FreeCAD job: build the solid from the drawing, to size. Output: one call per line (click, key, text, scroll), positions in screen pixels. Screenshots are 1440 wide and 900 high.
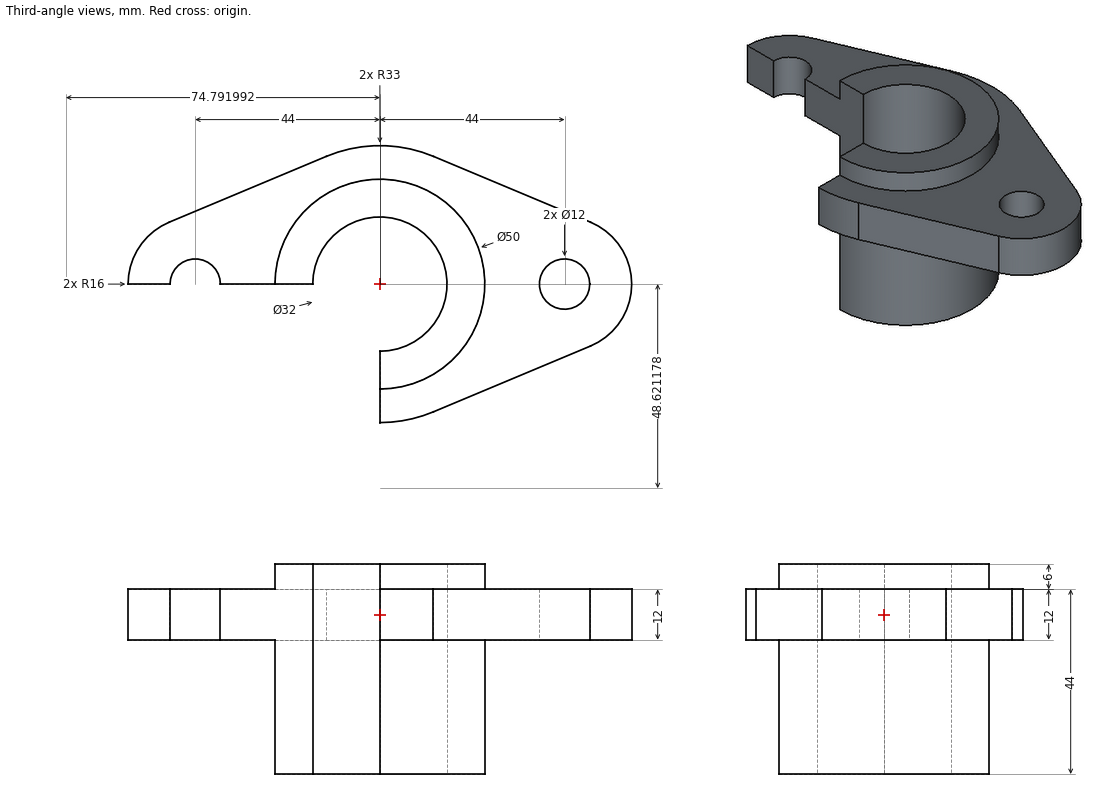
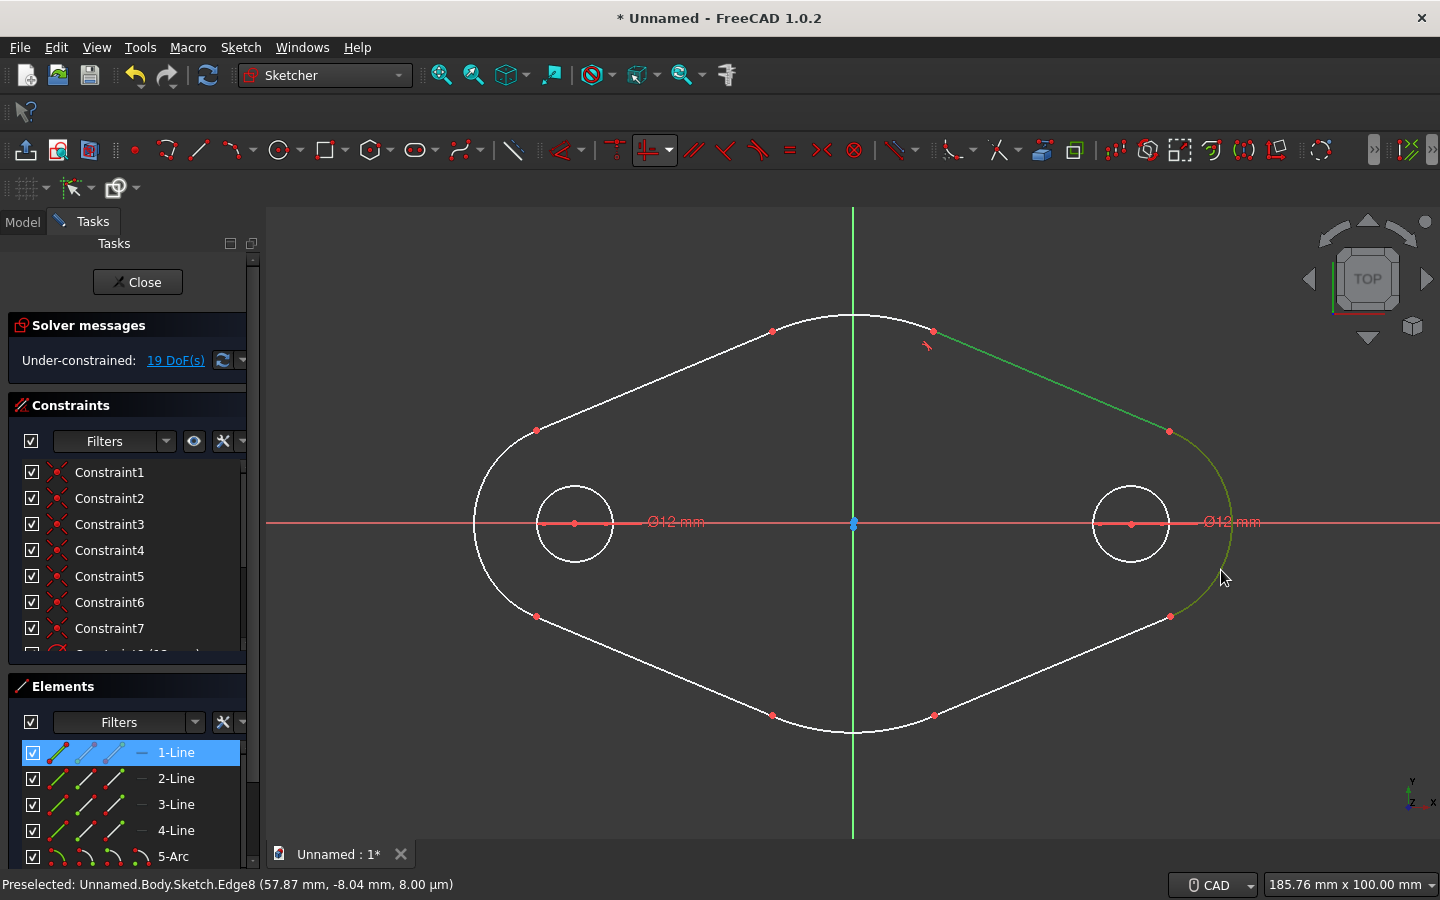
key(t)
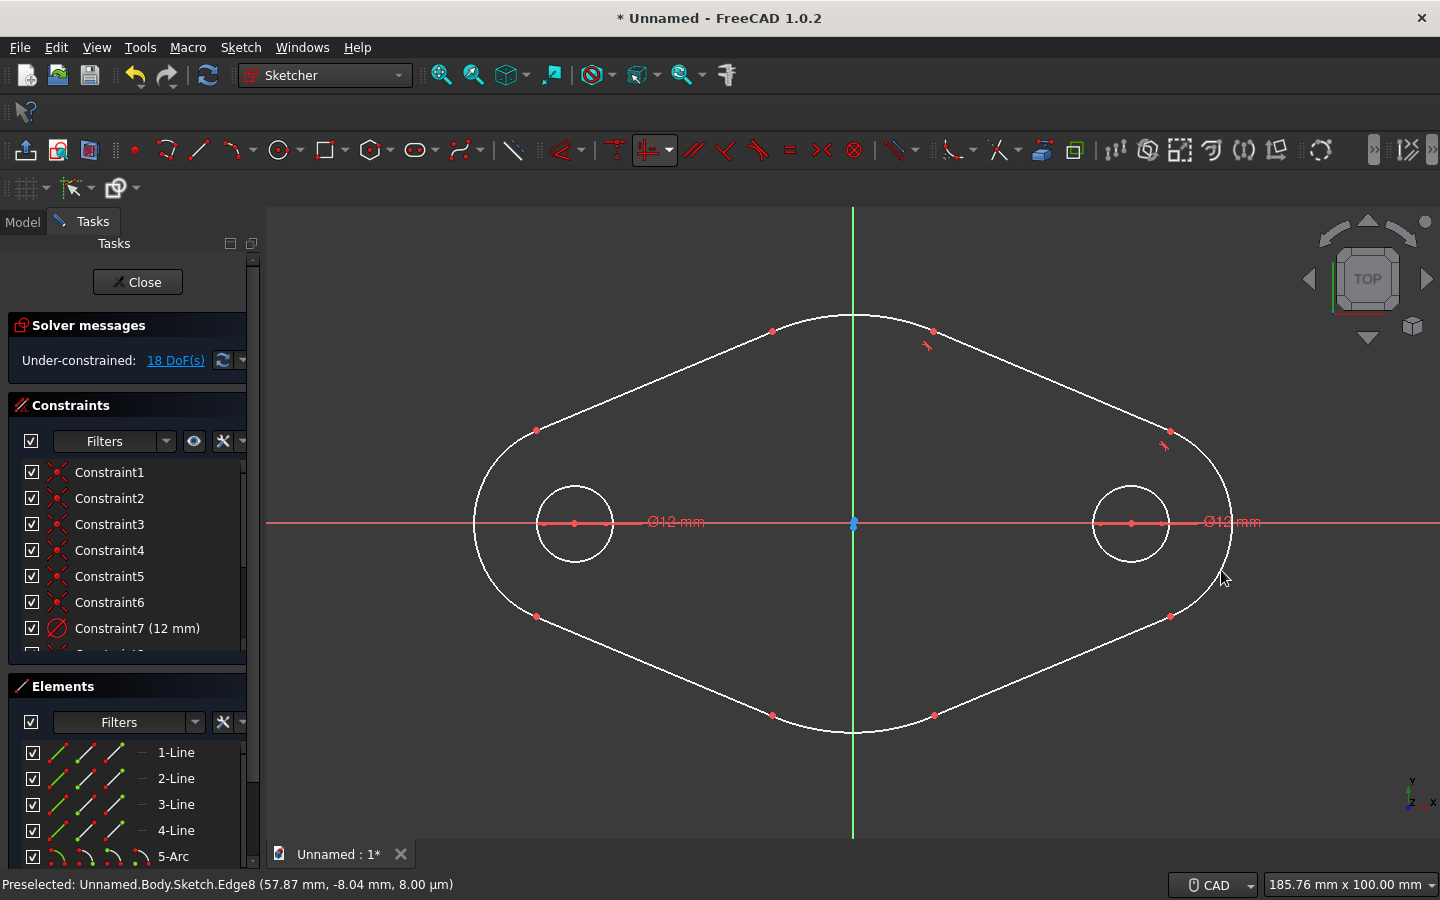
click(701, 362)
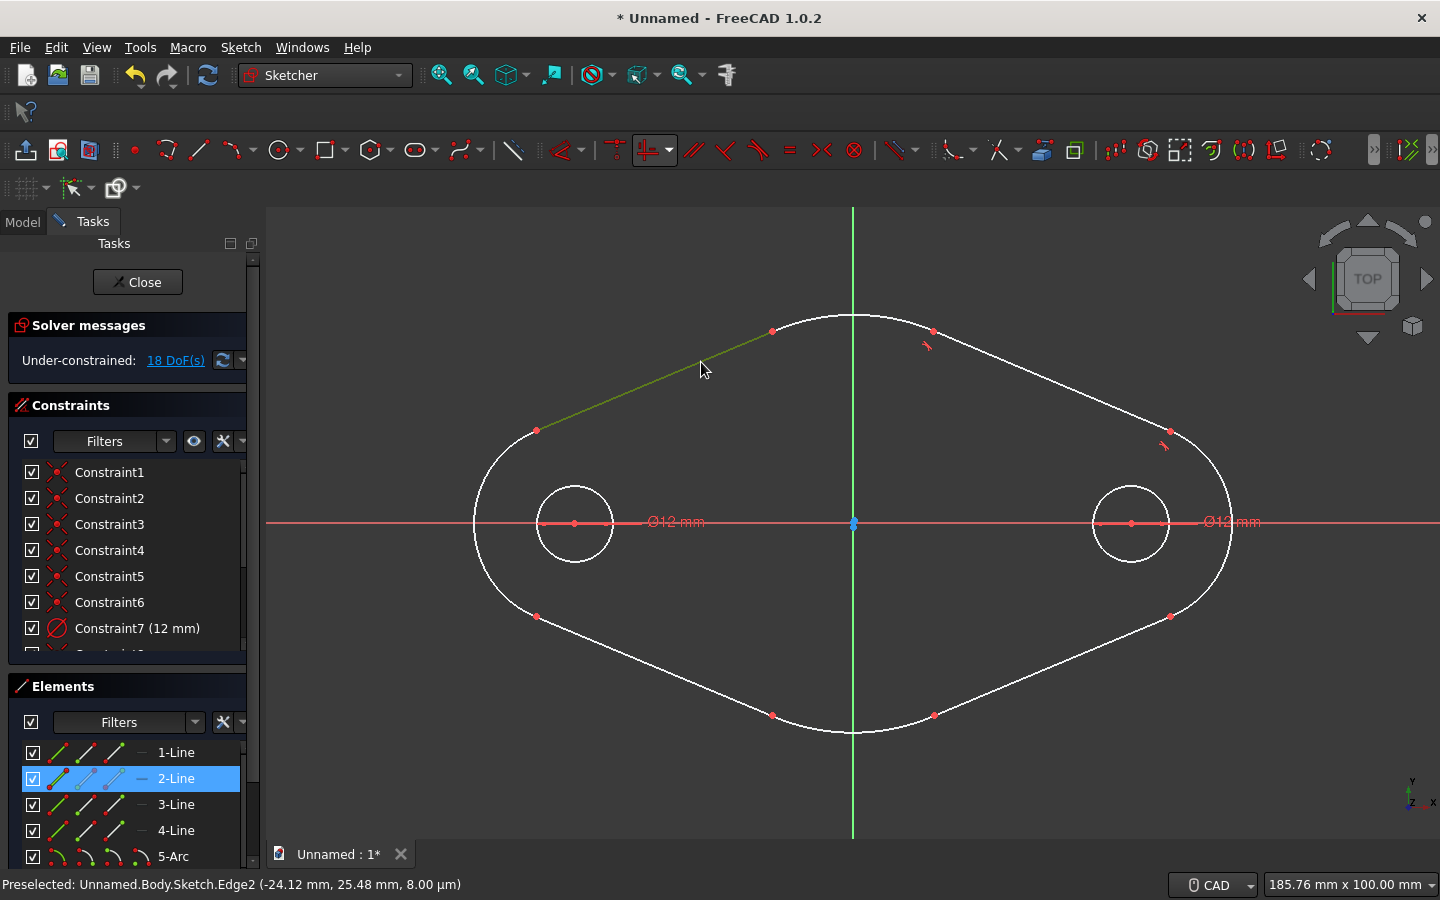
click(886, 317)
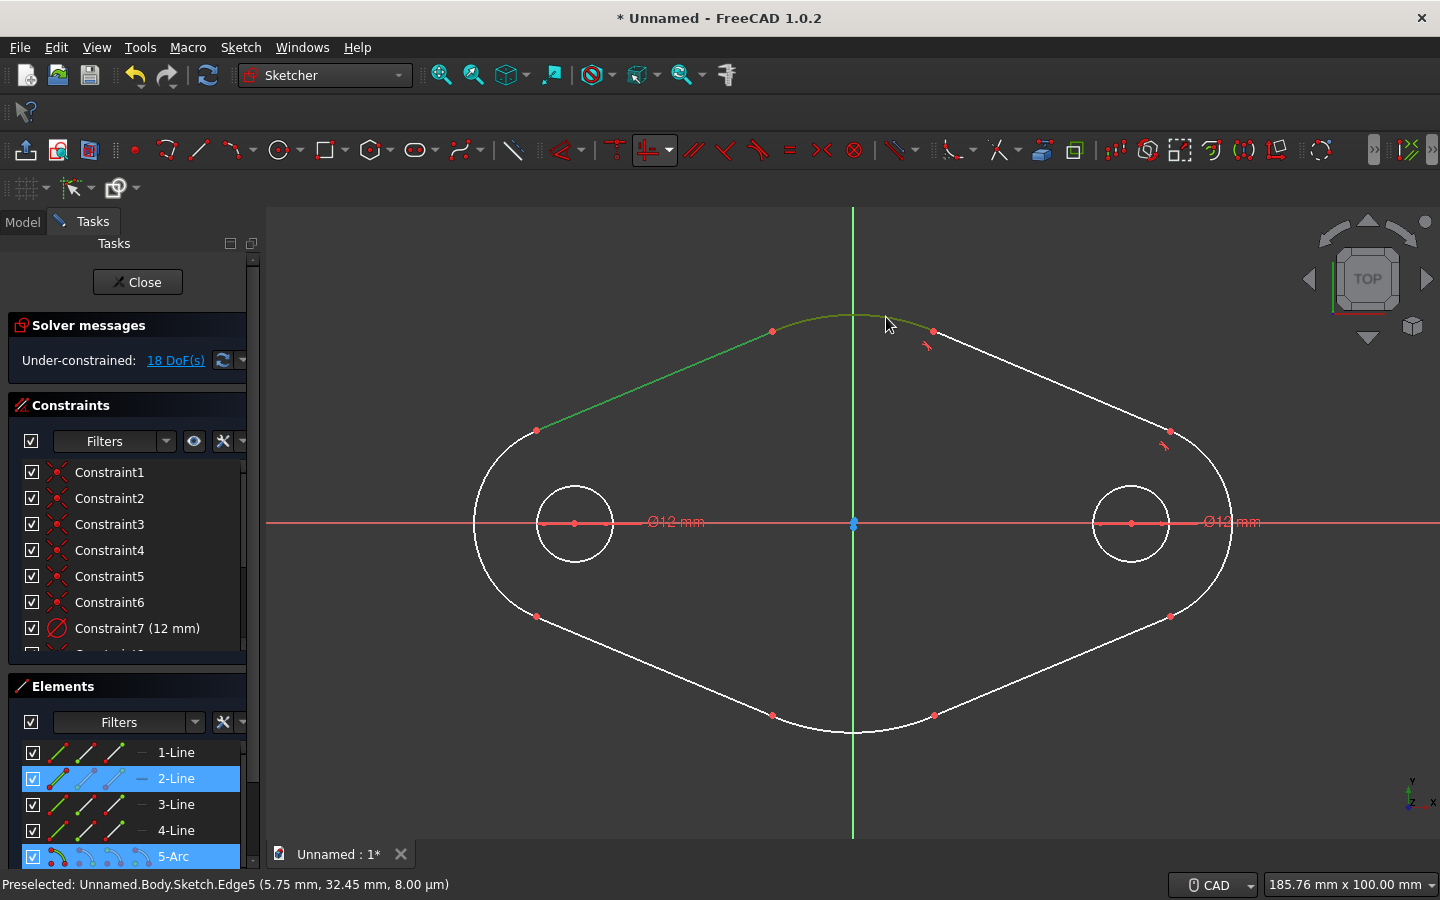
click(758, 150)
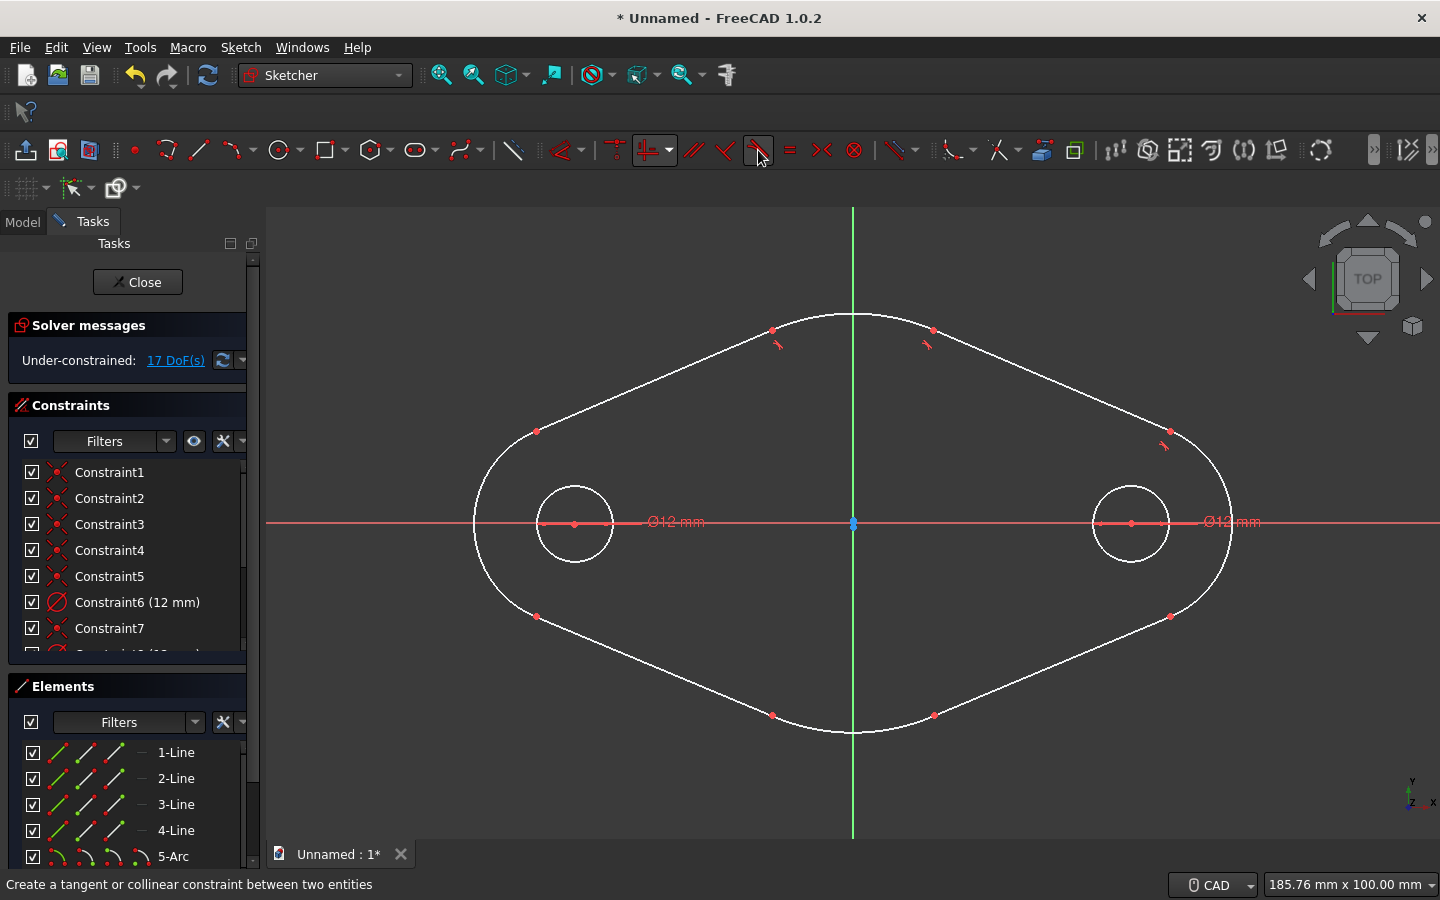
click(701, 360)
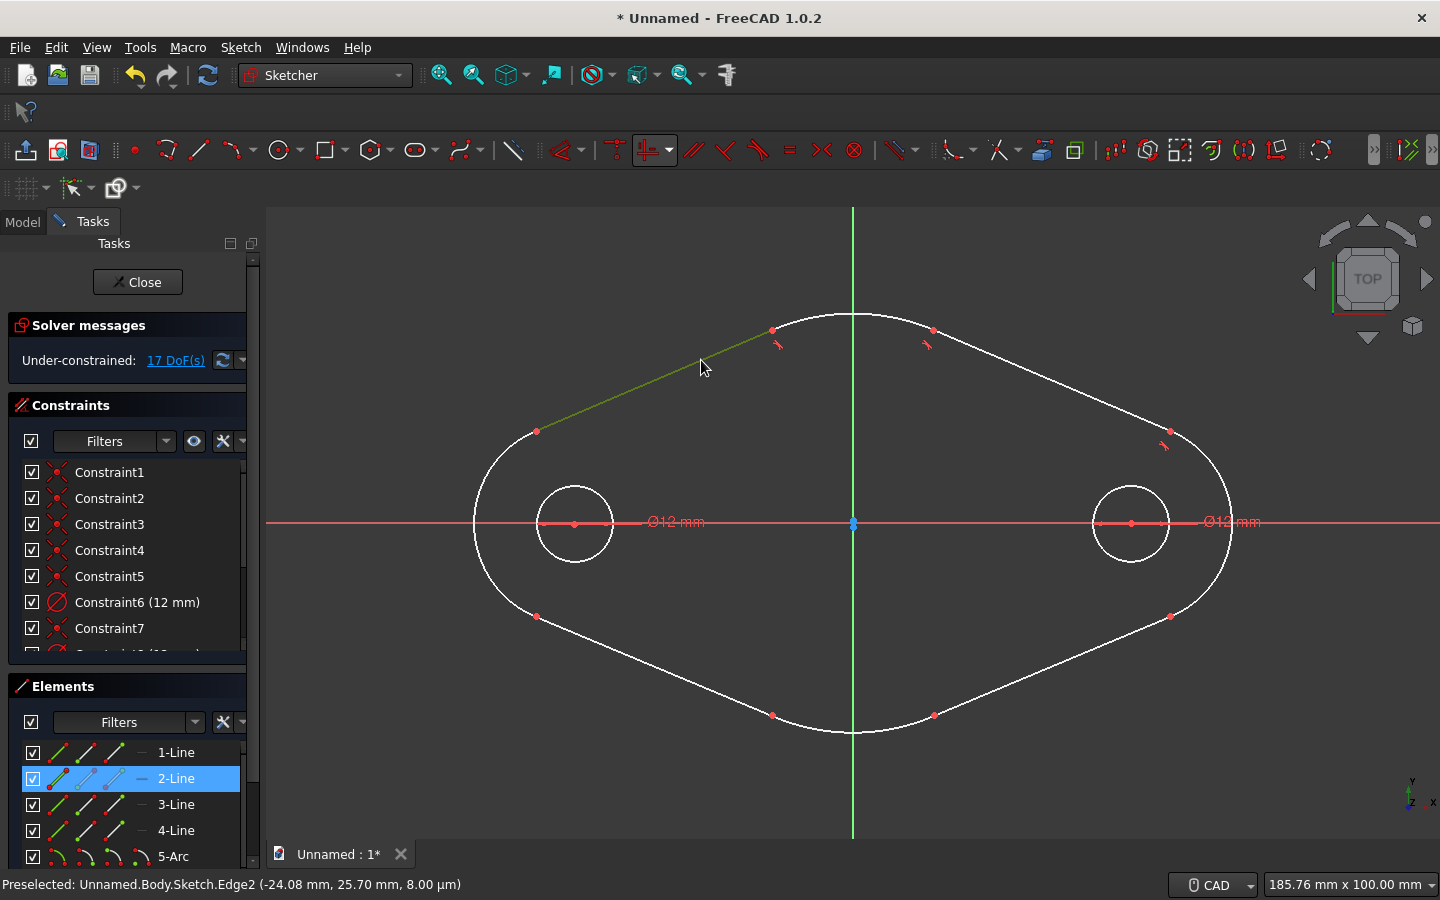
click(485, 478)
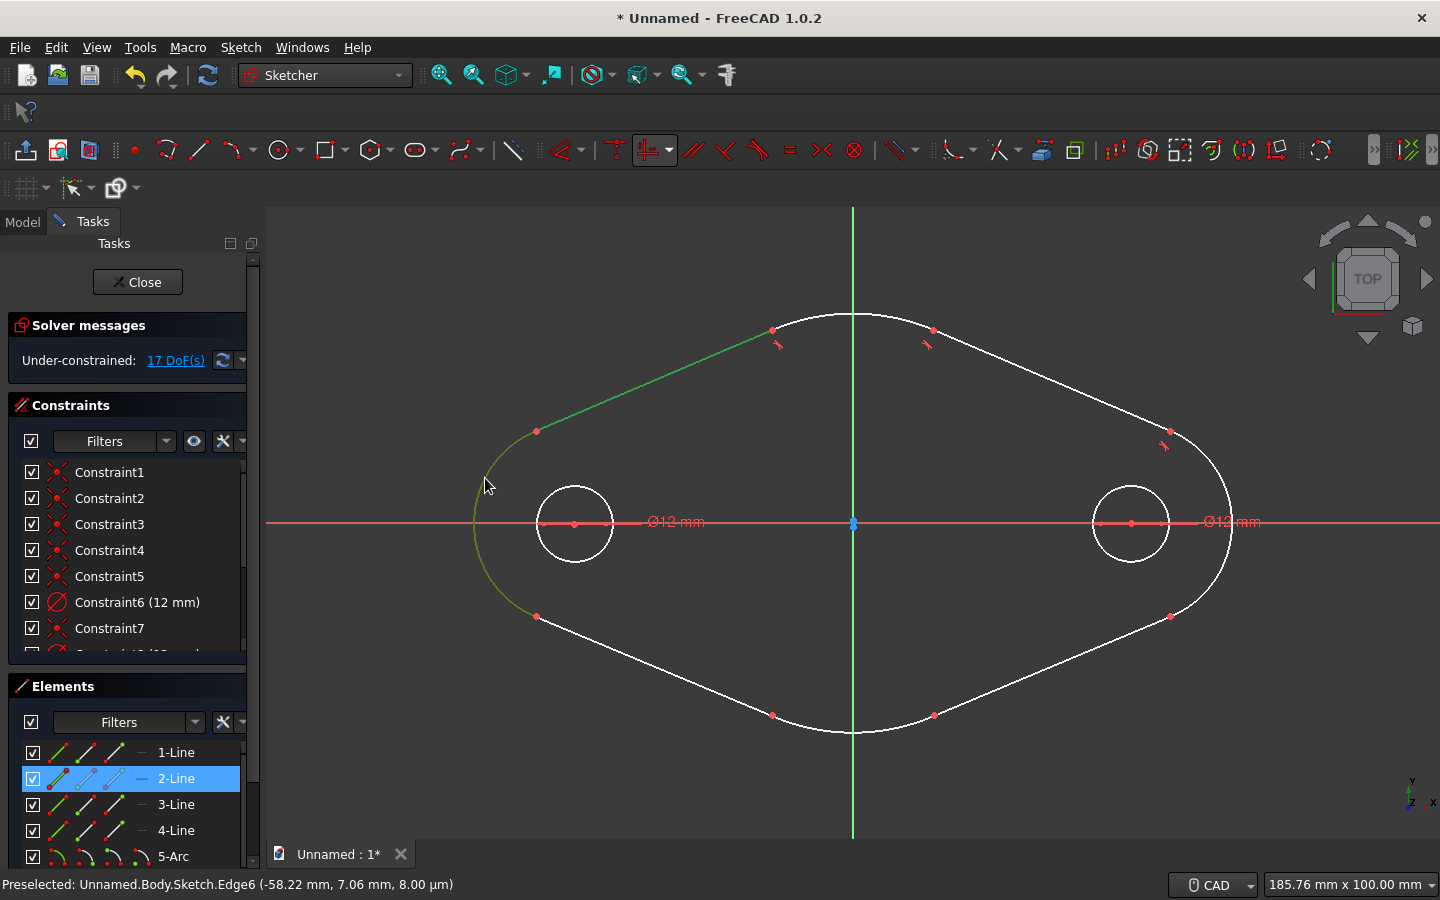
key(t)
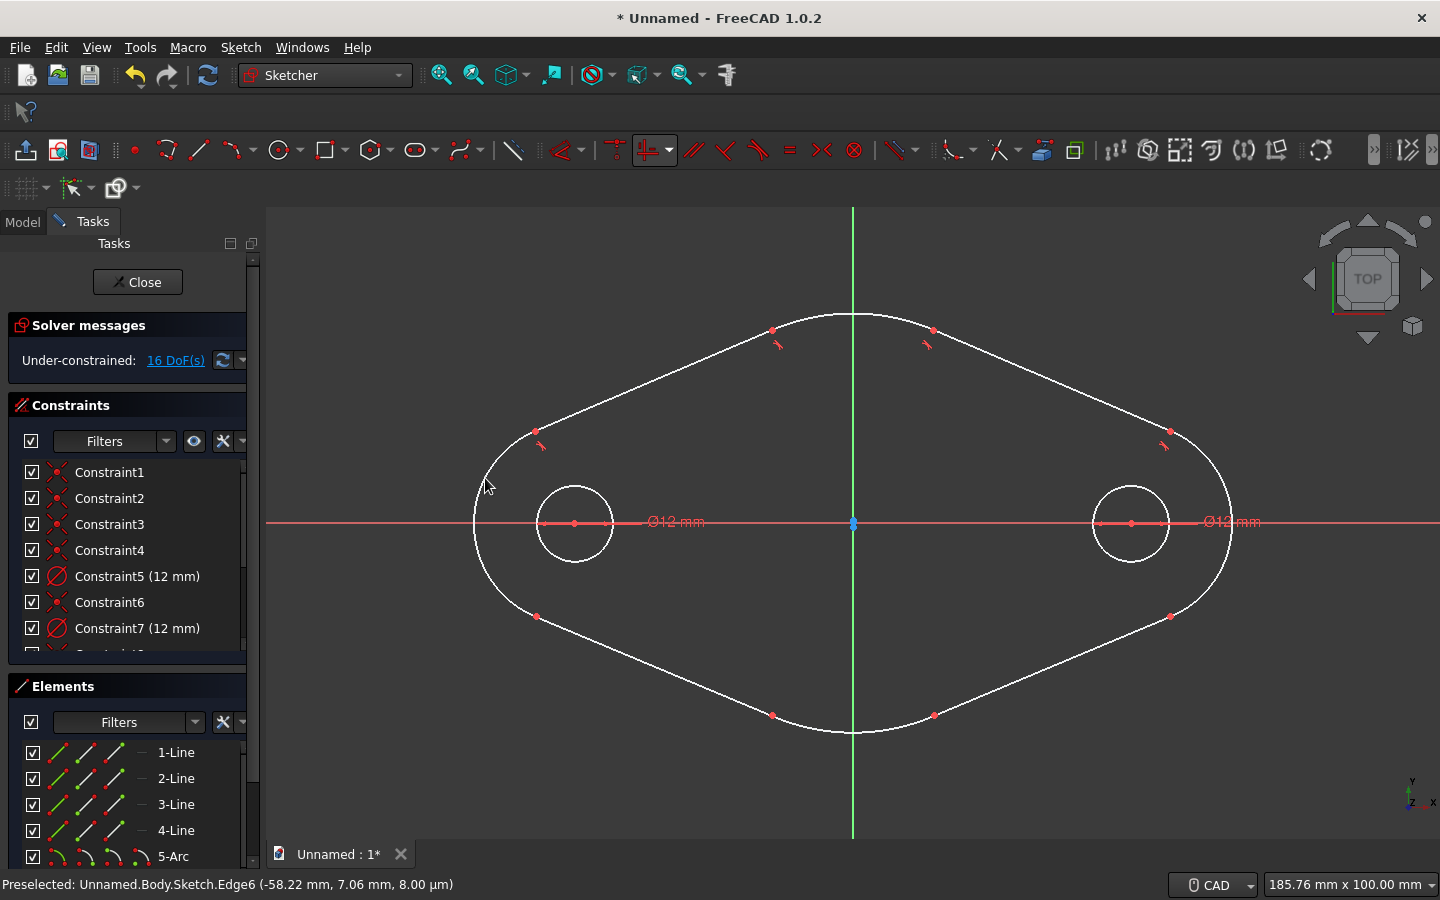
click(607, 647)